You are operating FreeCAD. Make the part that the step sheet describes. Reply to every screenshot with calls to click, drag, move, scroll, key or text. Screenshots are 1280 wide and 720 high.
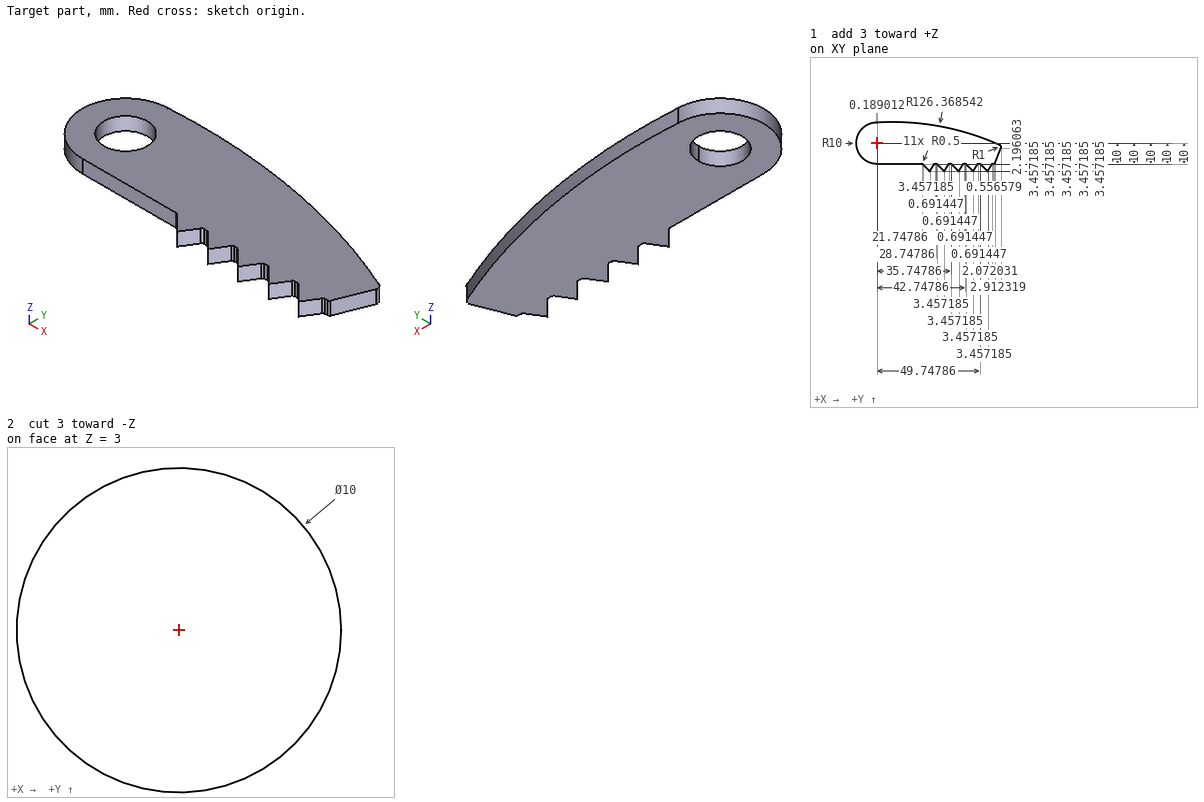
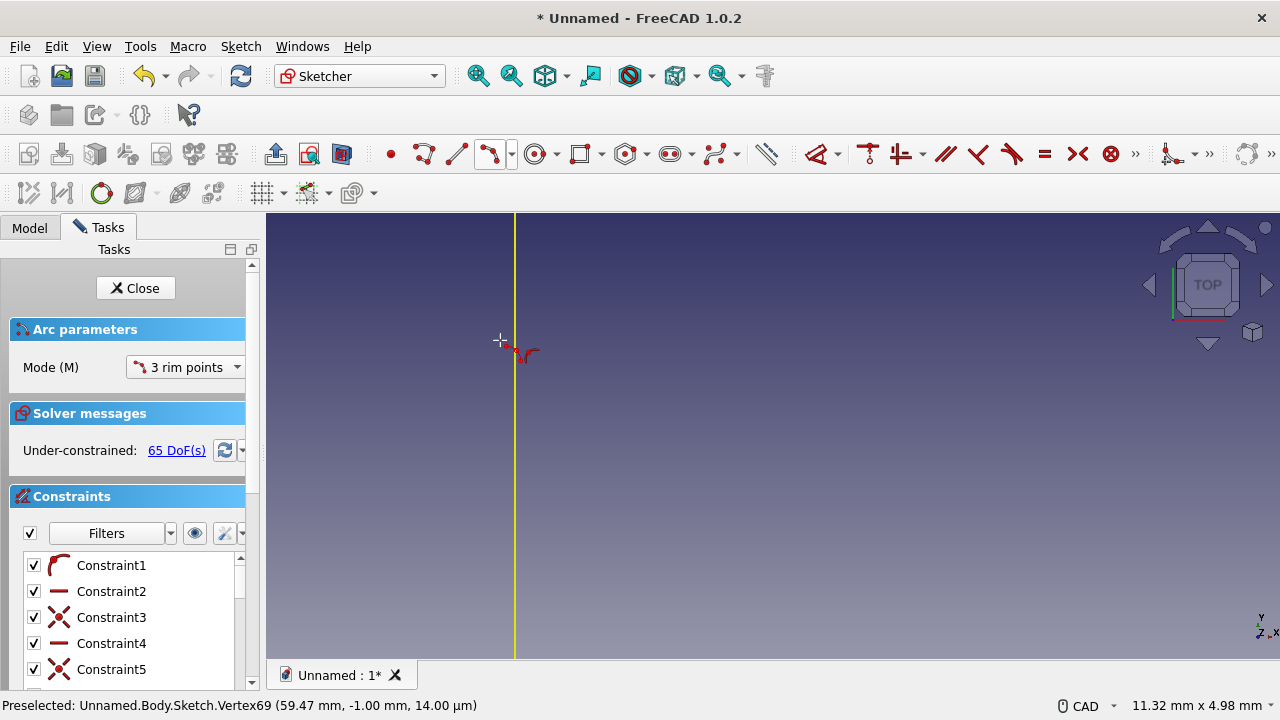
click(499, 341)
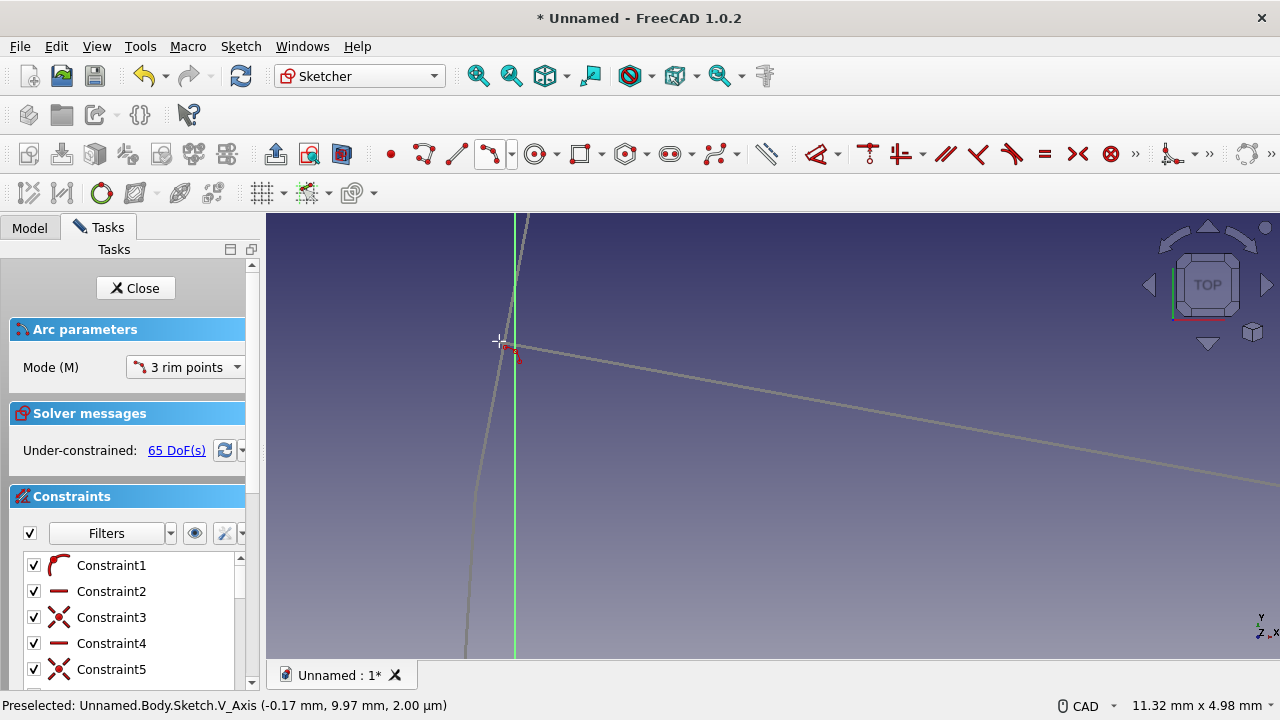
scroll(500, 340, down, 12)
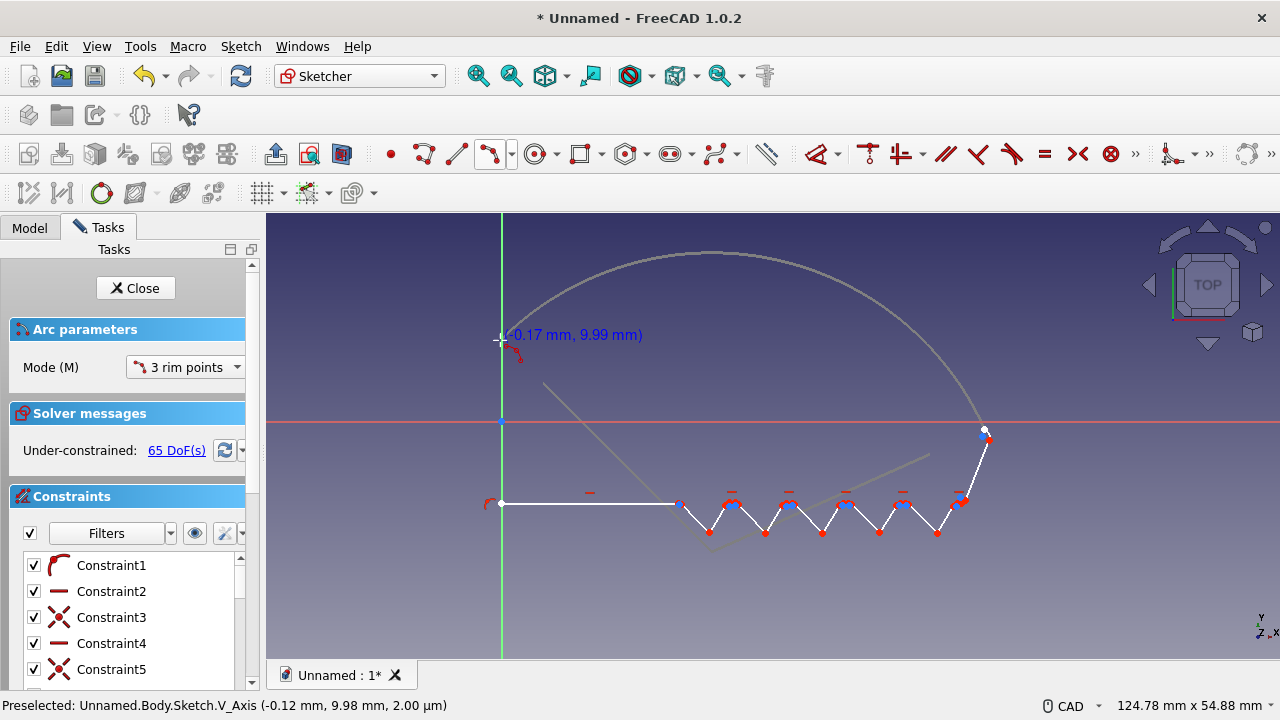
click(748, 355)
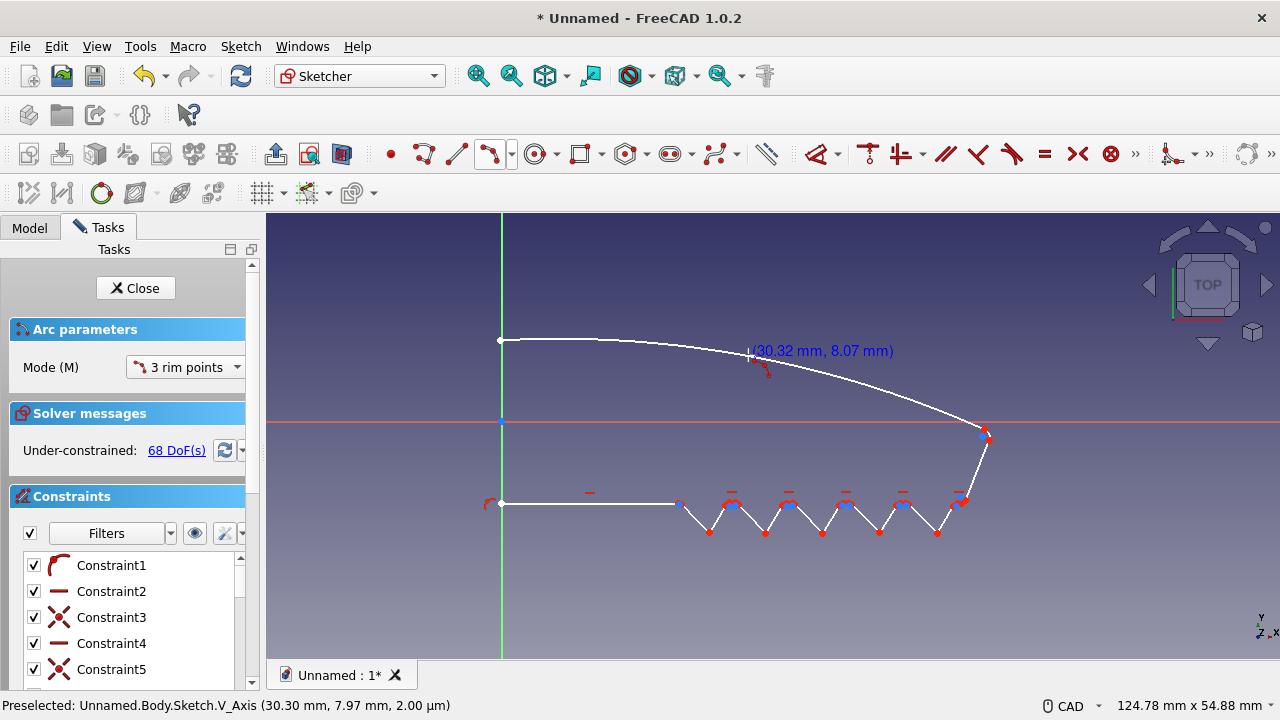
scroll(500, 340, up, 12)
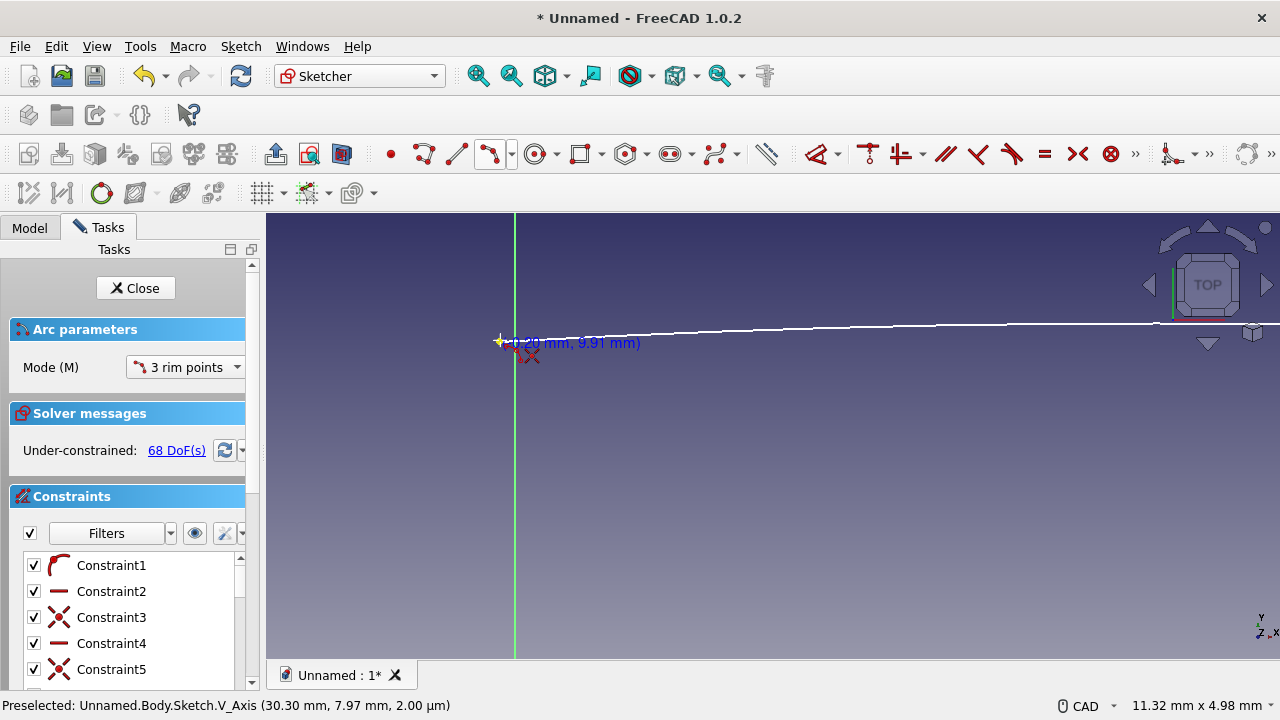
click(499, 342)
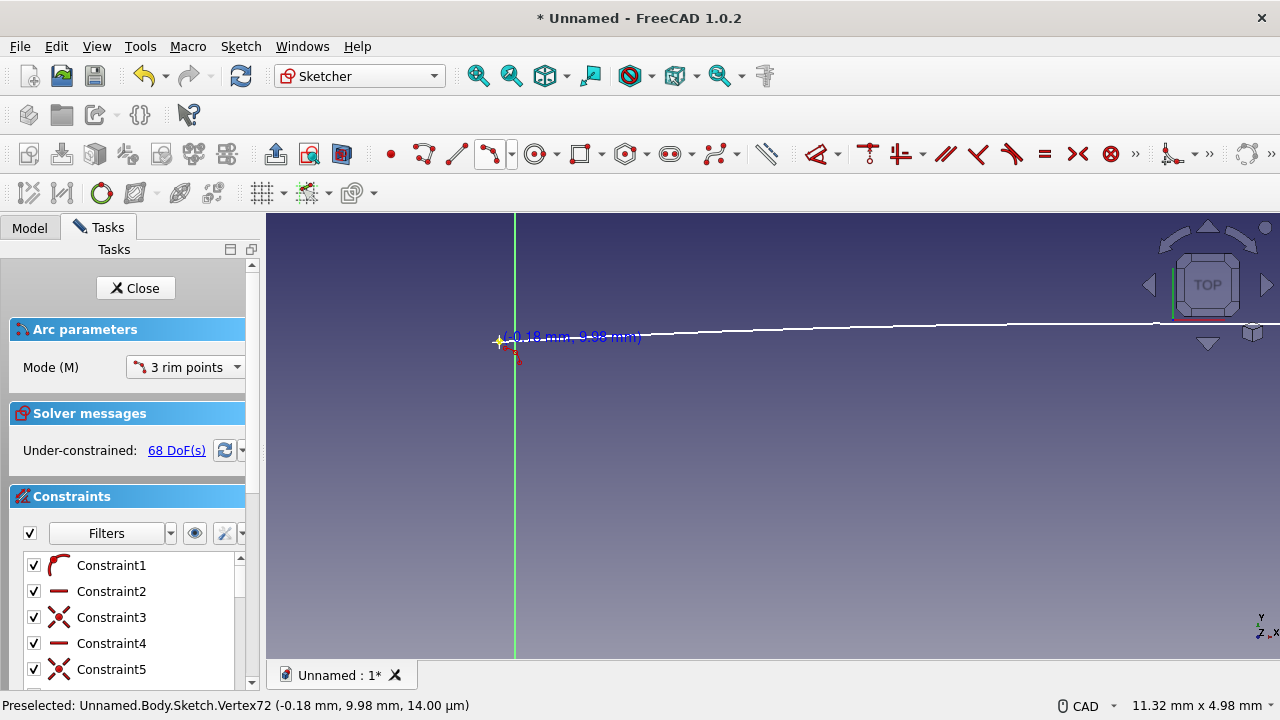
scroll(500, 340, down, 12)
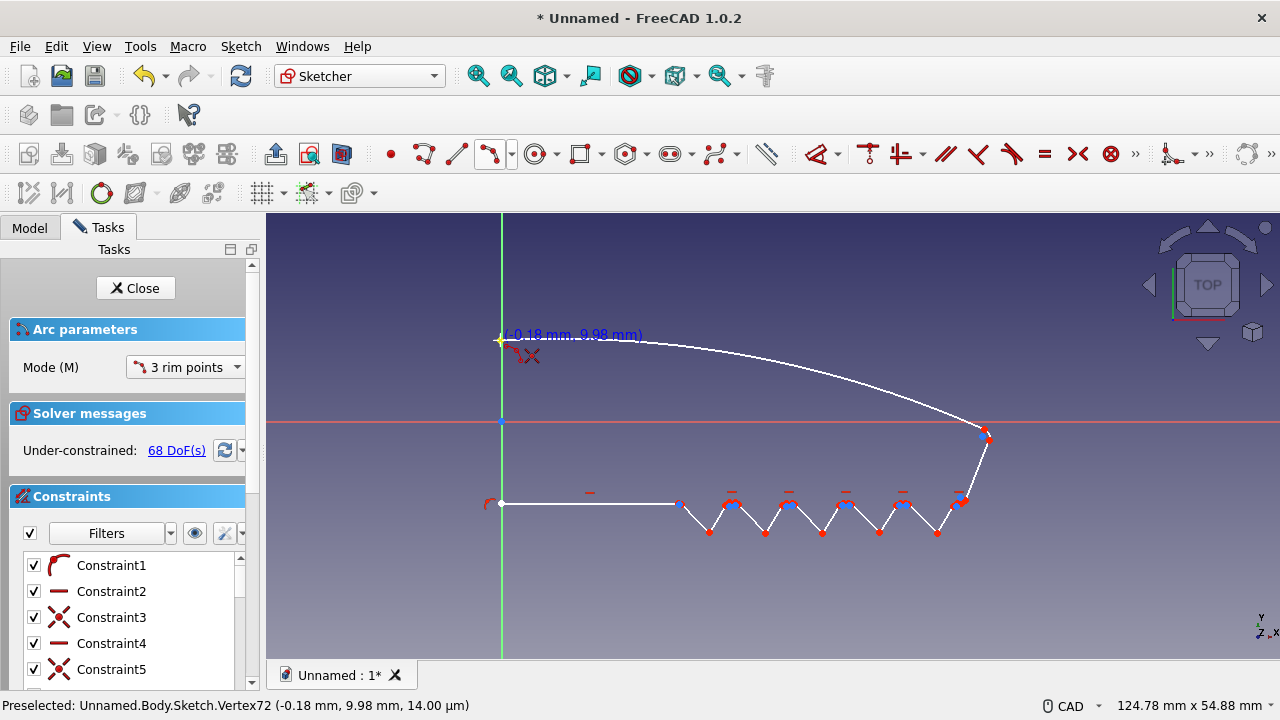
click(502, 504)
click(424, 397)
key(Escape)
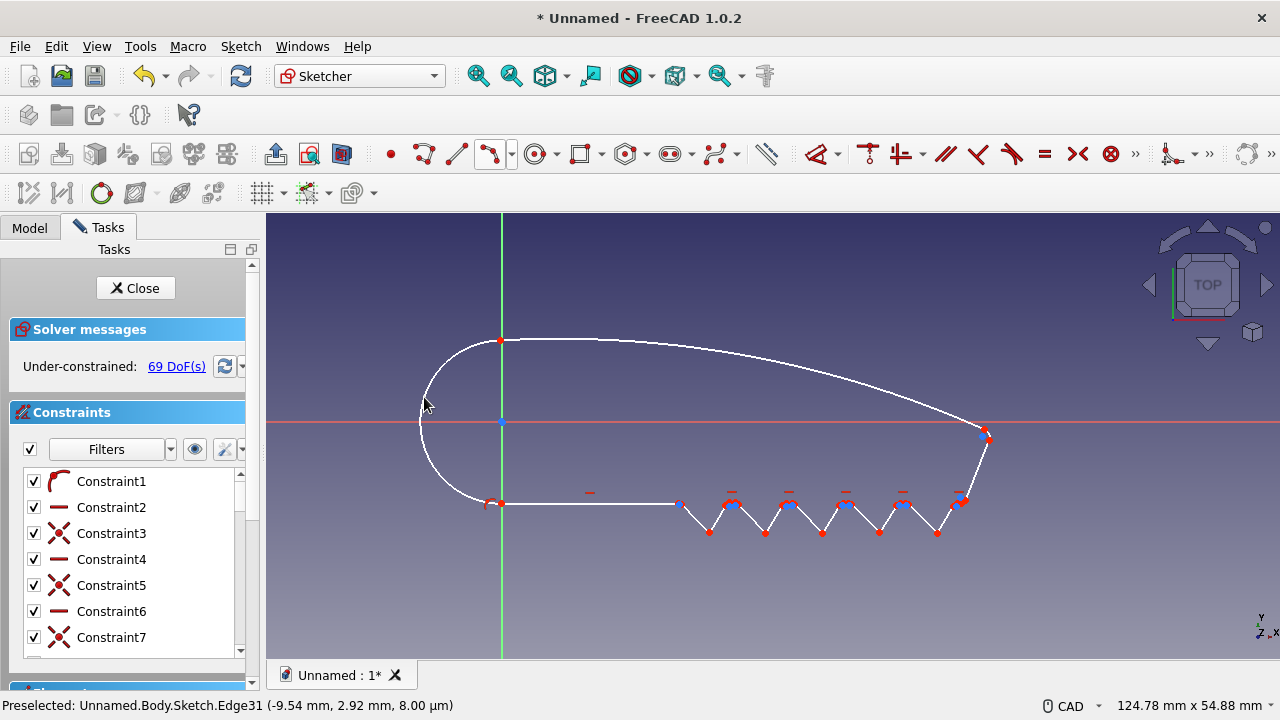
click(555, 504)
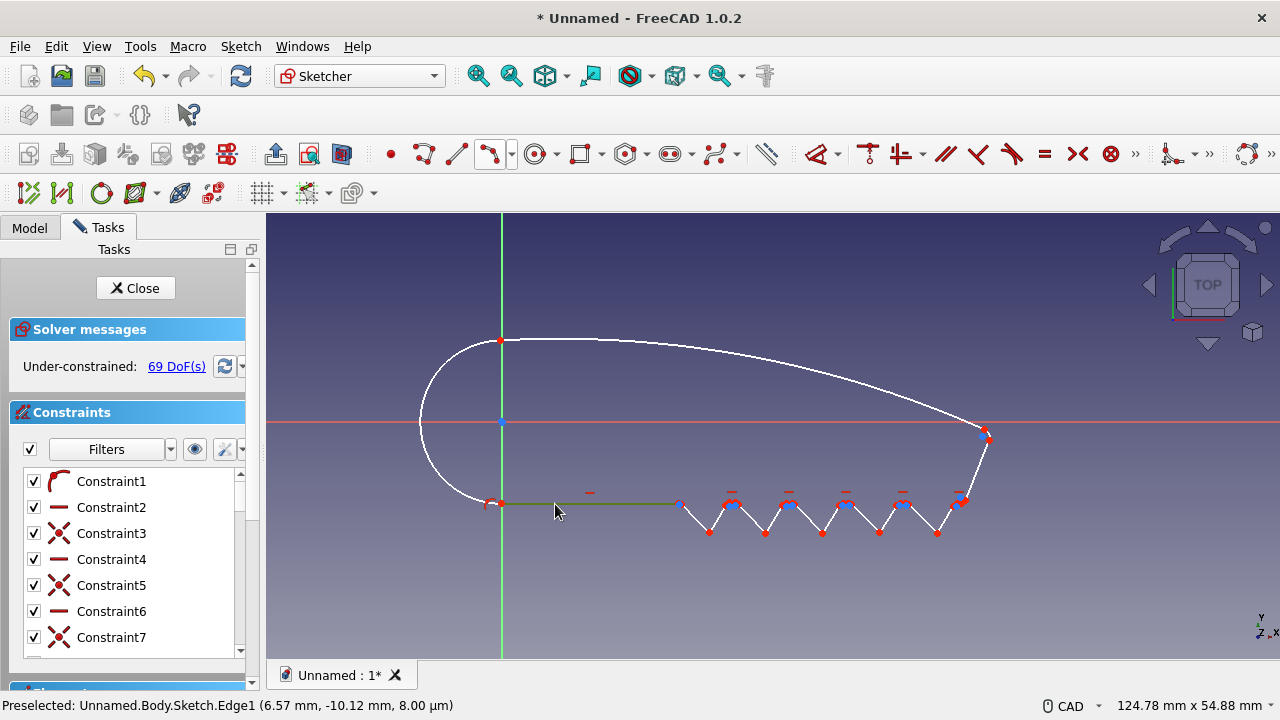
scroll(680, 503, up, 12)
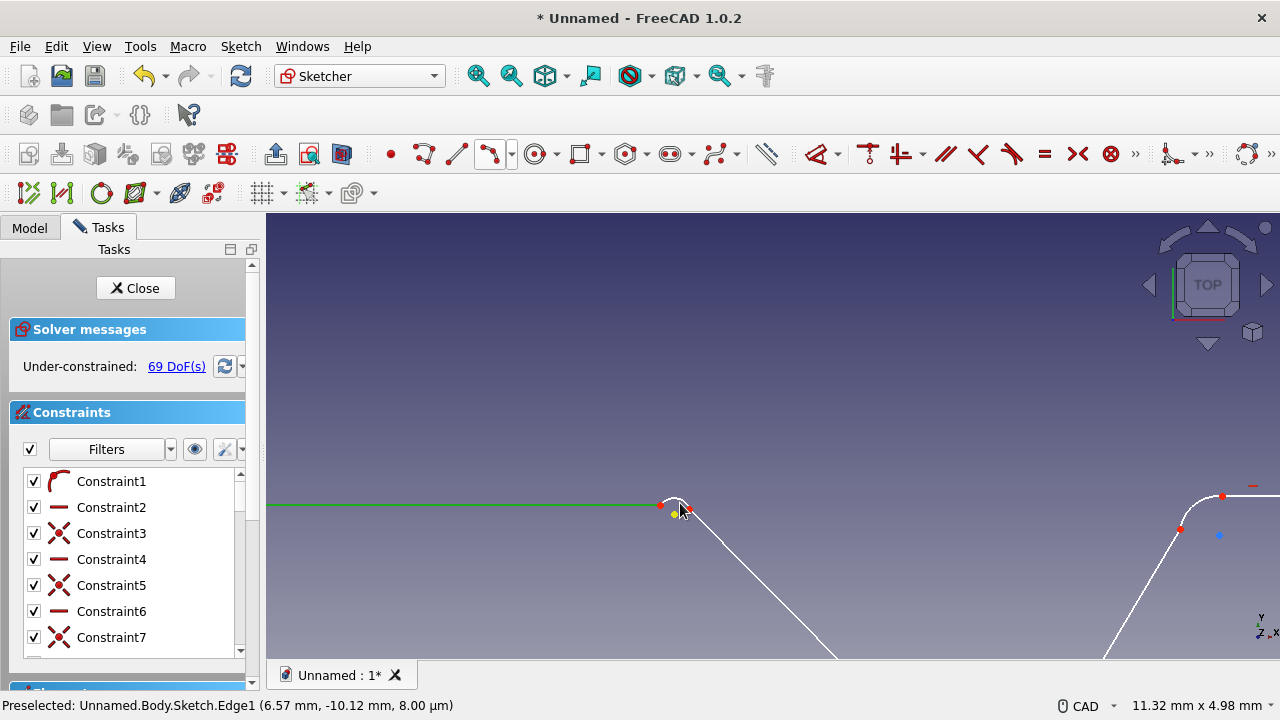
click(676, 498)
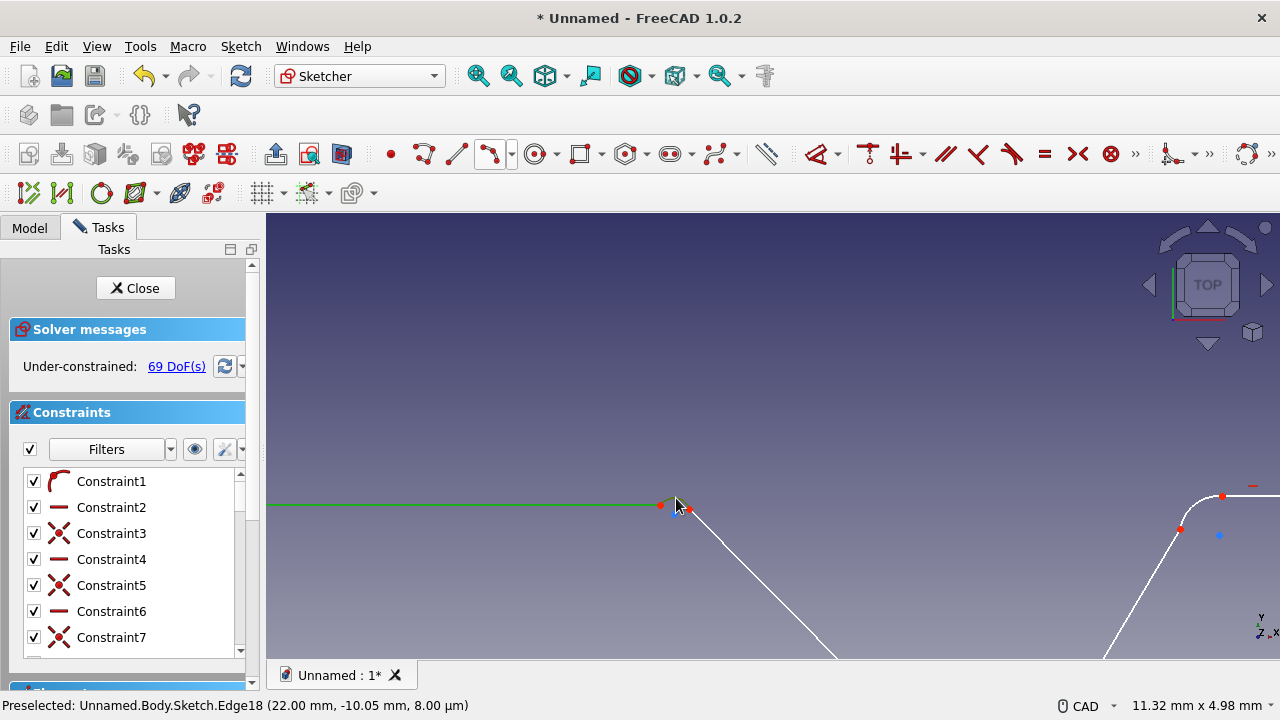
key(t)